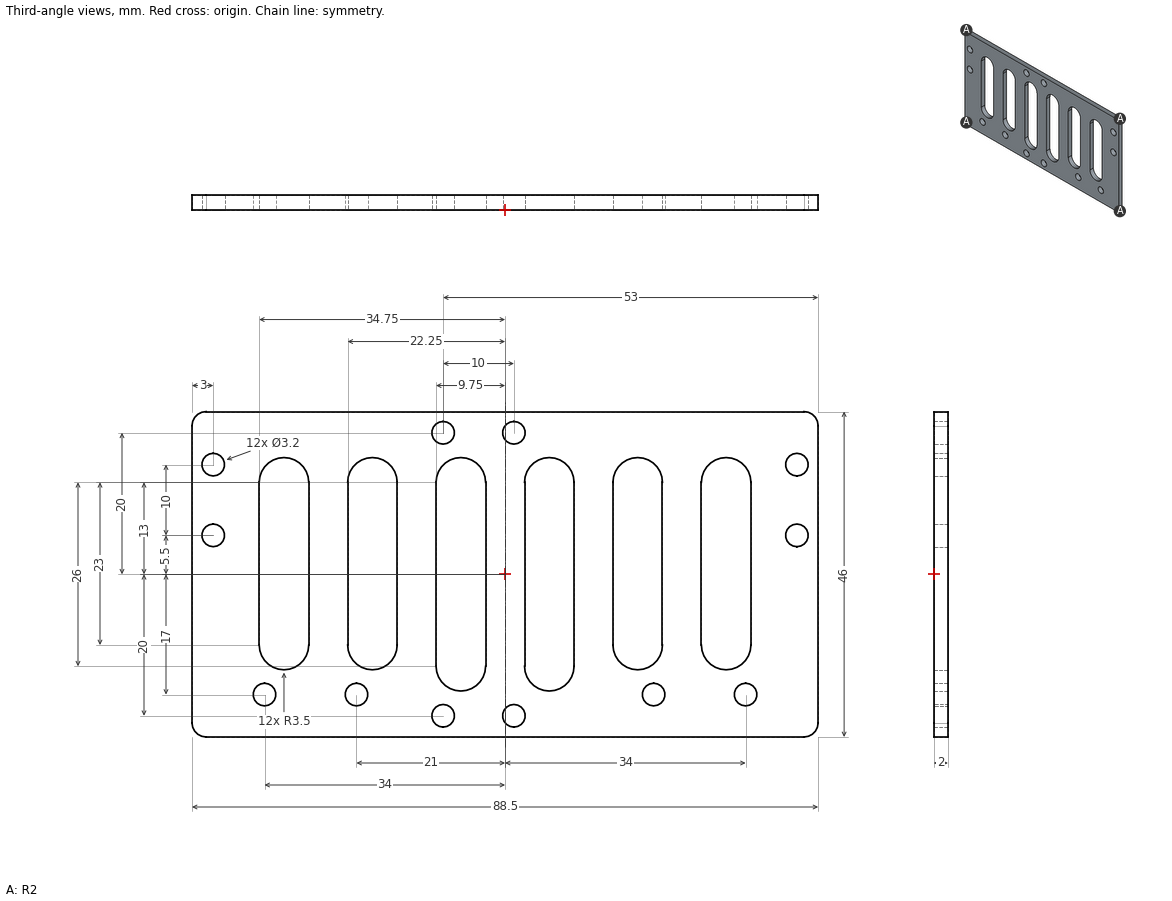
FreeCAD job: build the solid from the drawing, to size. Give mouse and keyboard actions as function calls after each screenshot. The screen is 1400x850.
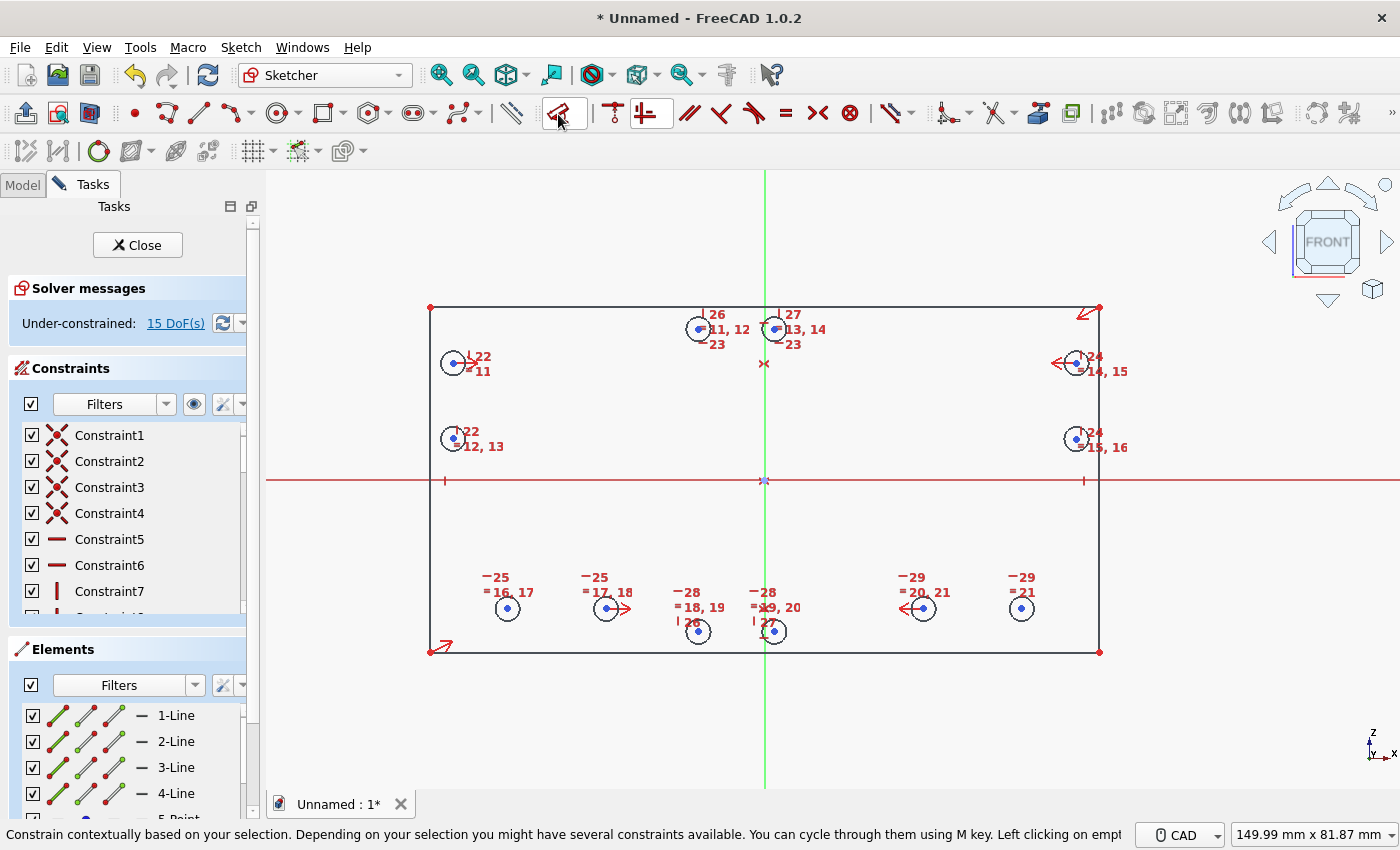
scroll(462, 355, up, 3)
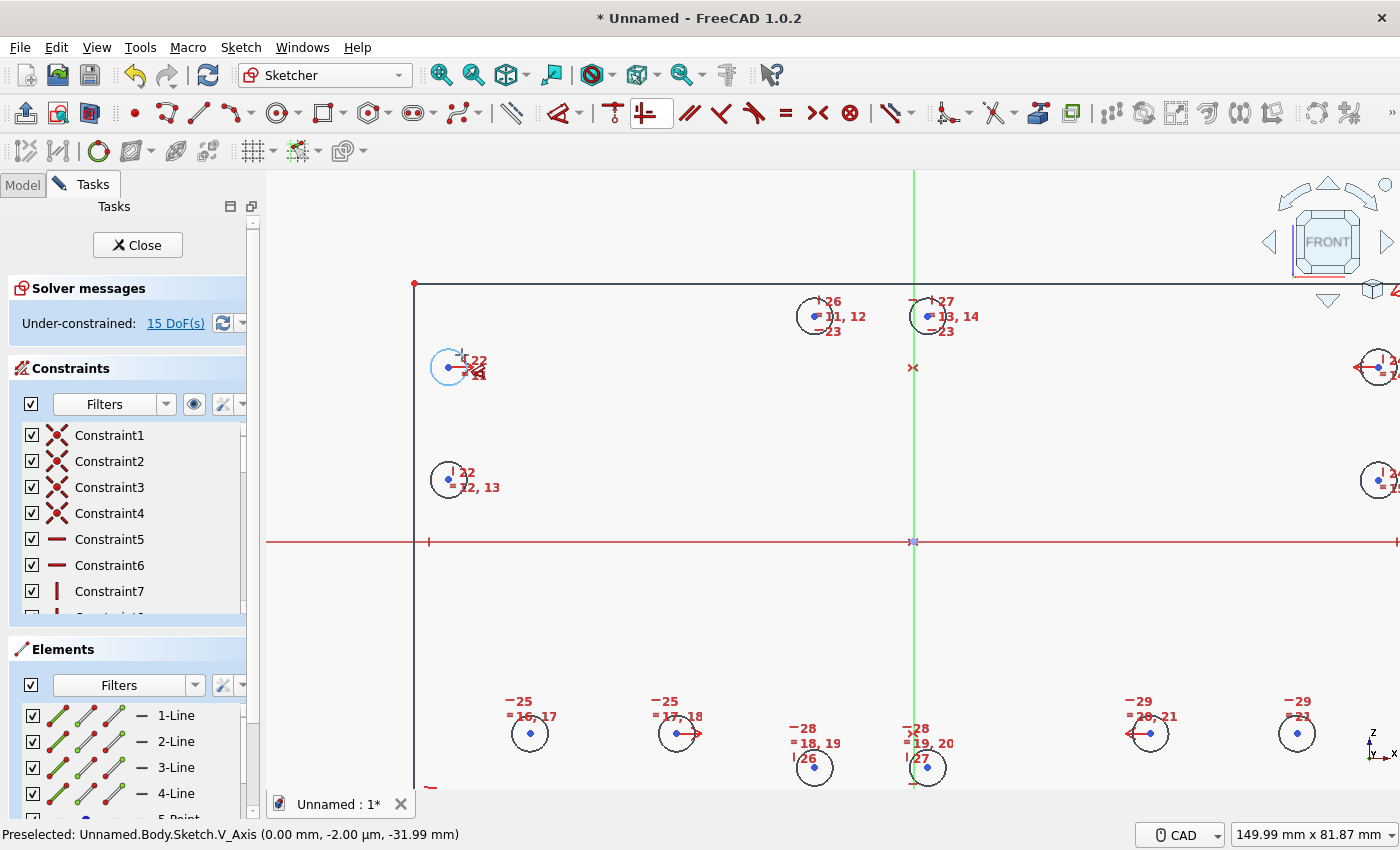
click(461, 354)
click(483, 331)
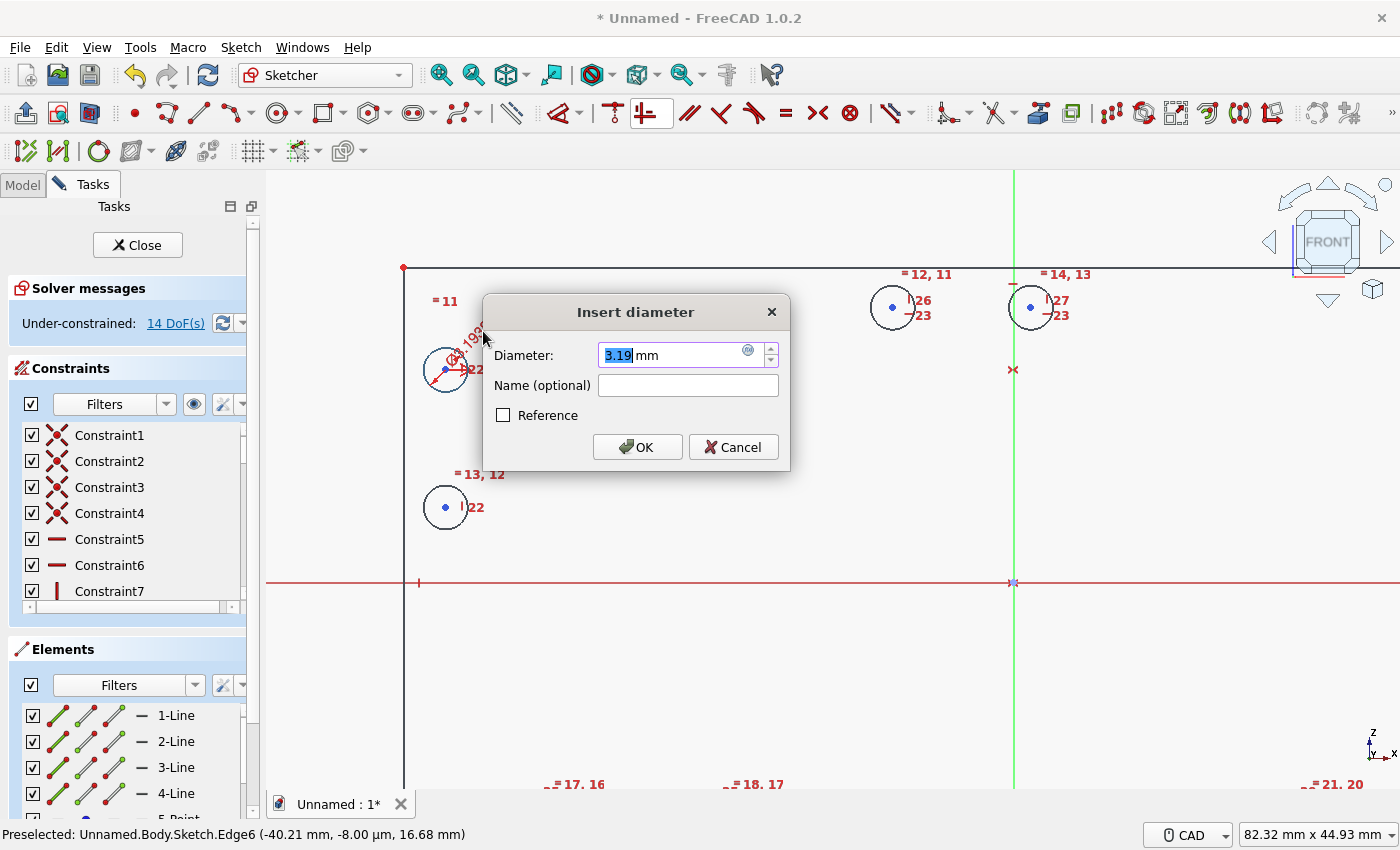
text(3.2)
key(Return)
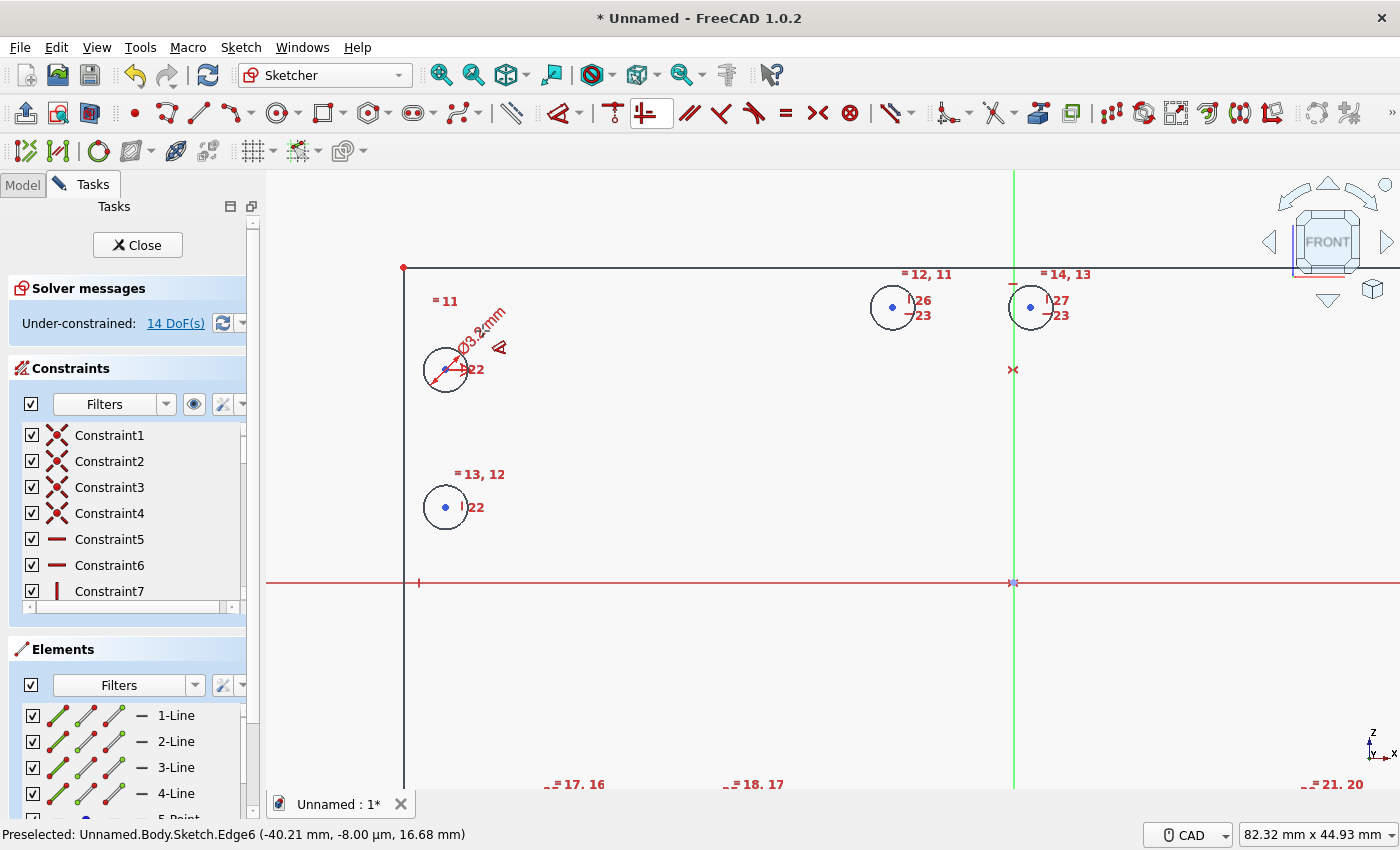
scroll(461, 354, down, 3)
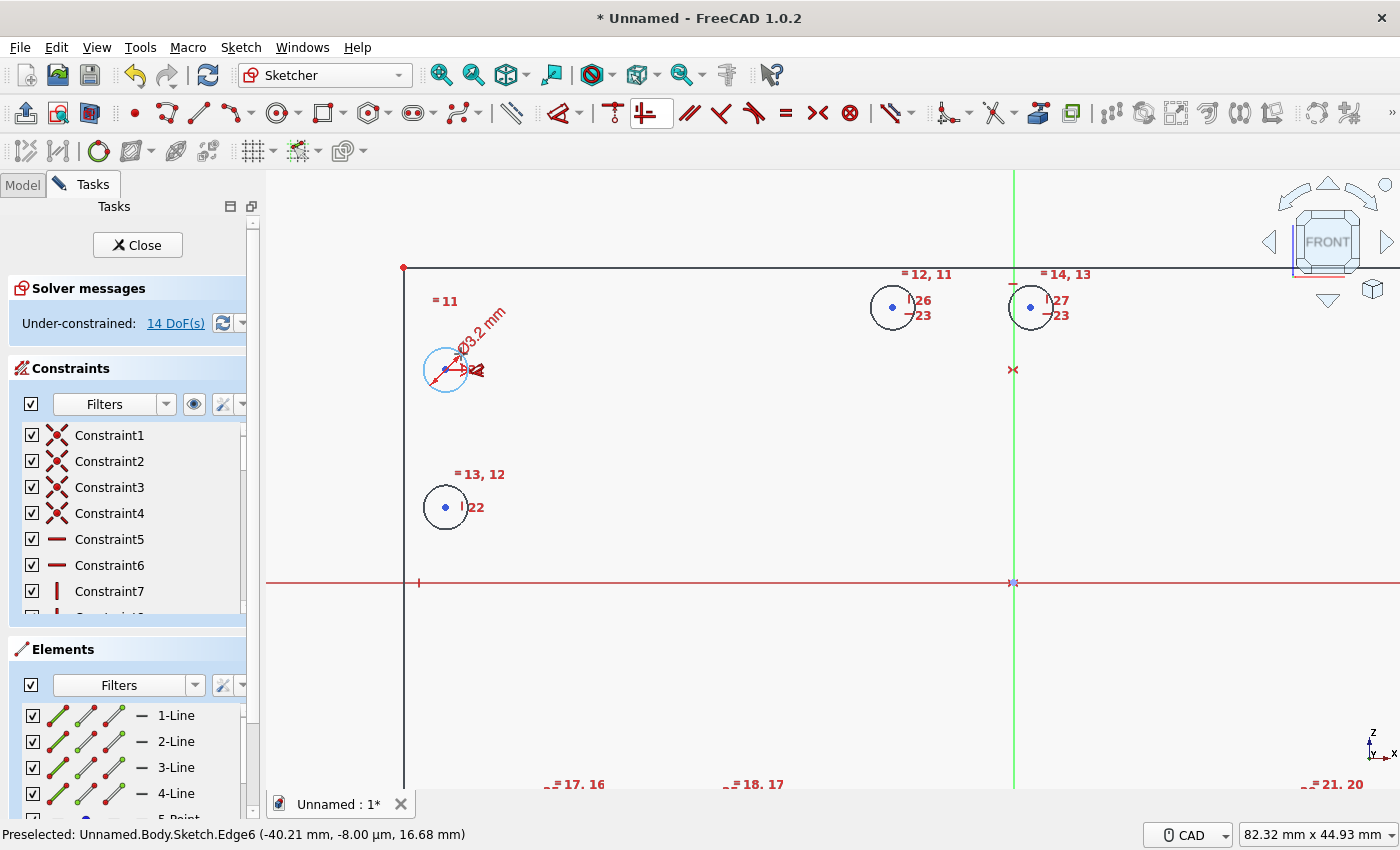
click(1099, 549)
click(1133, 400)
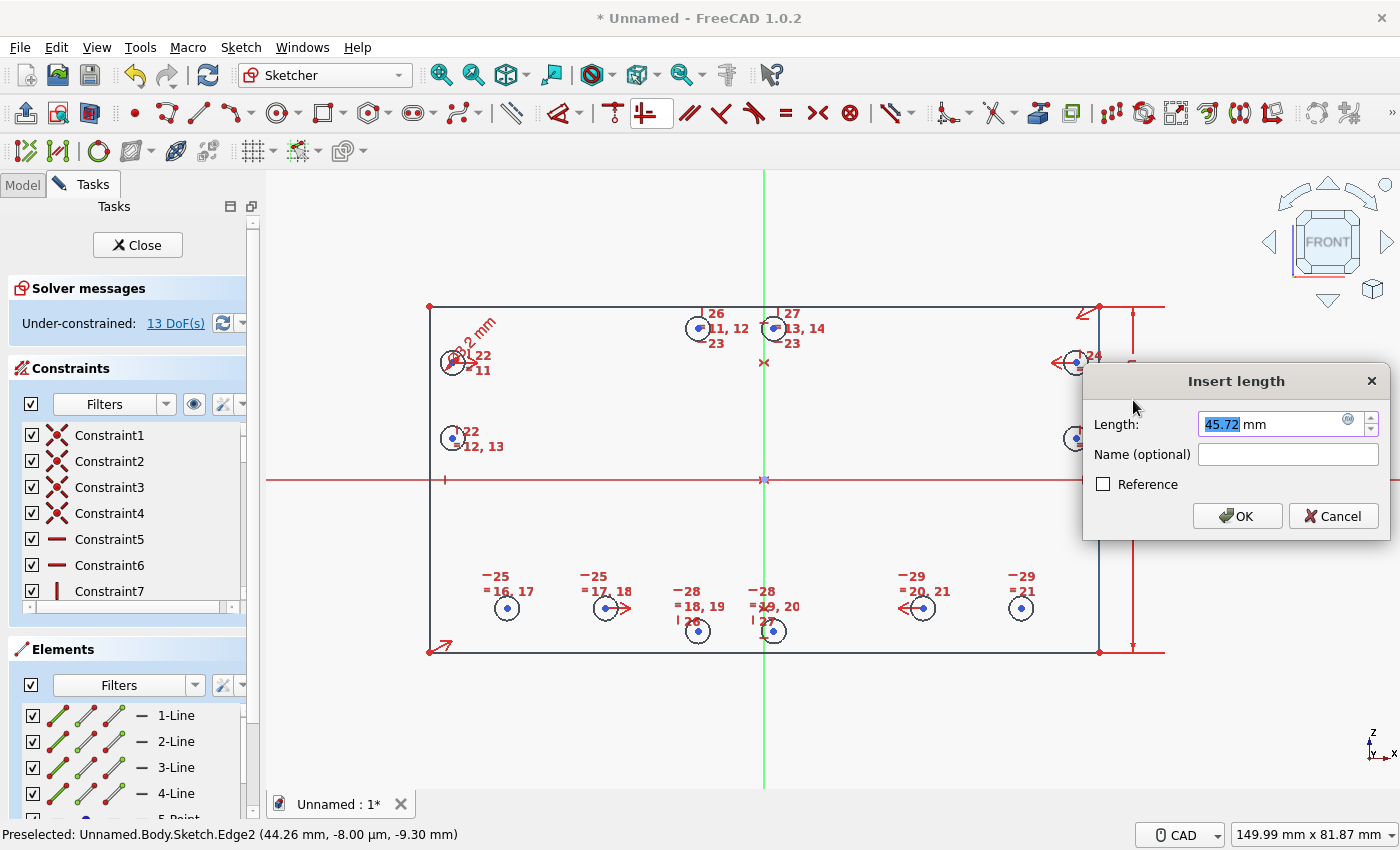
text(46)
key(Return)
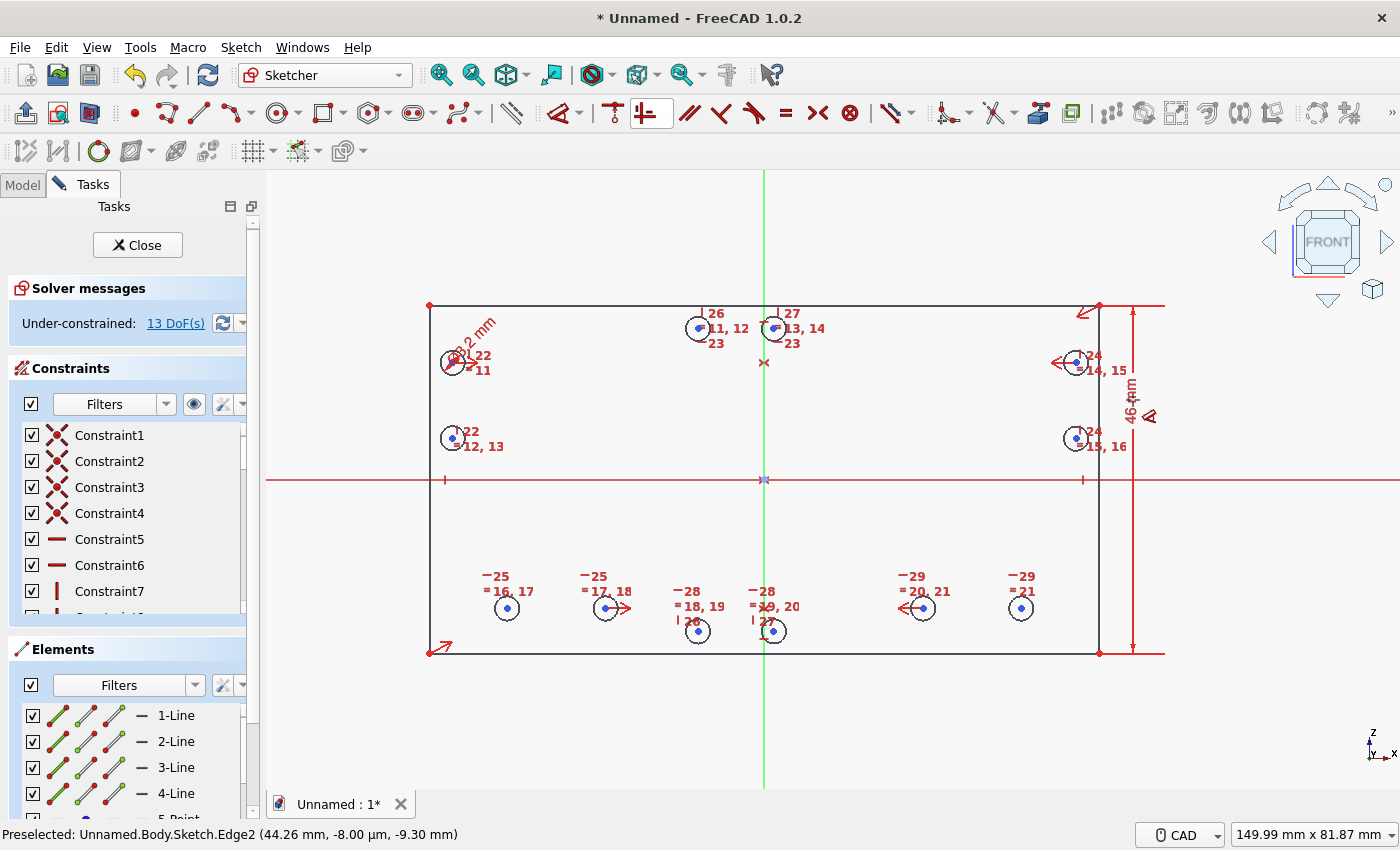
click(698, 329)
click(664, 404)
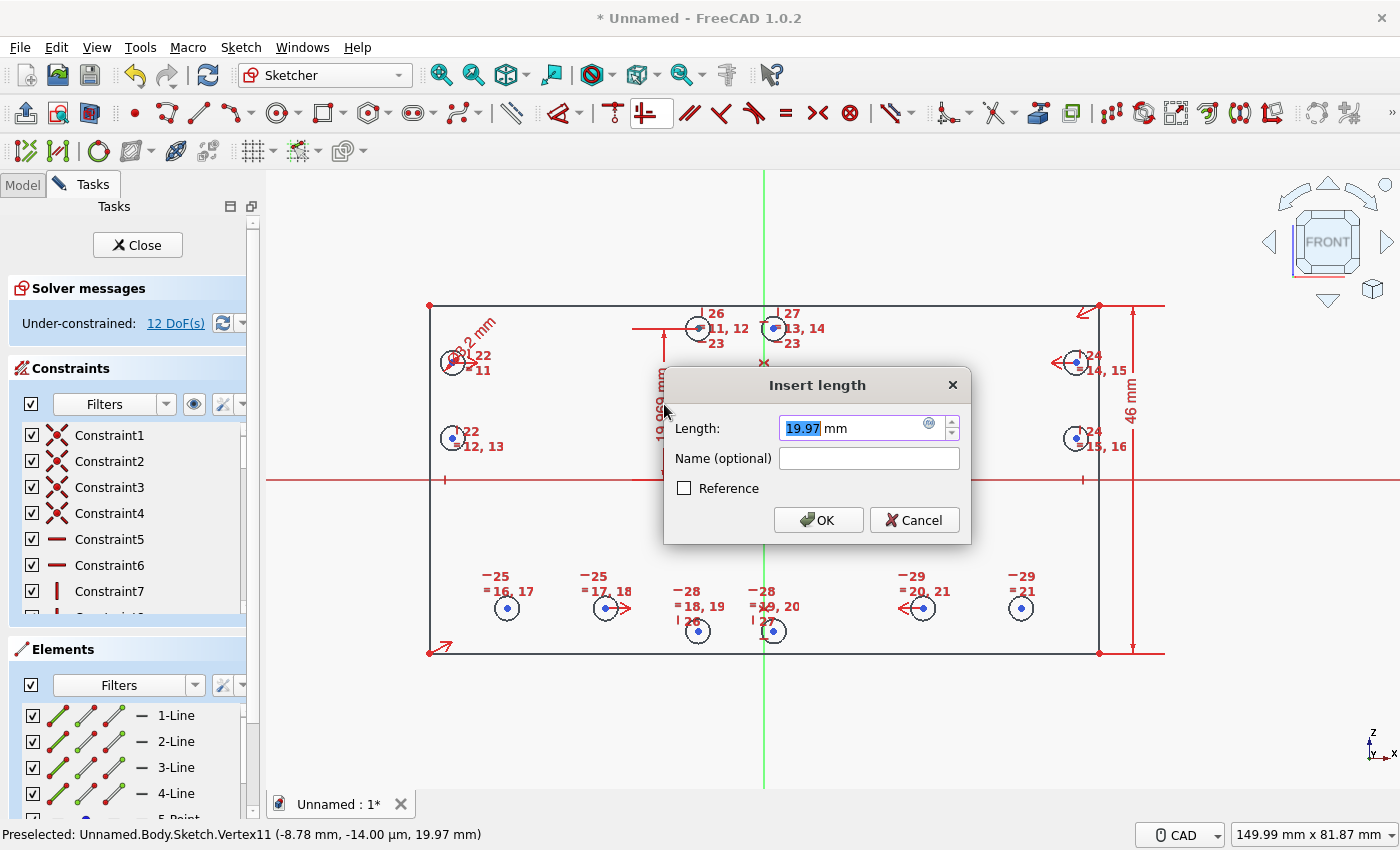
text(20)
key(Return)